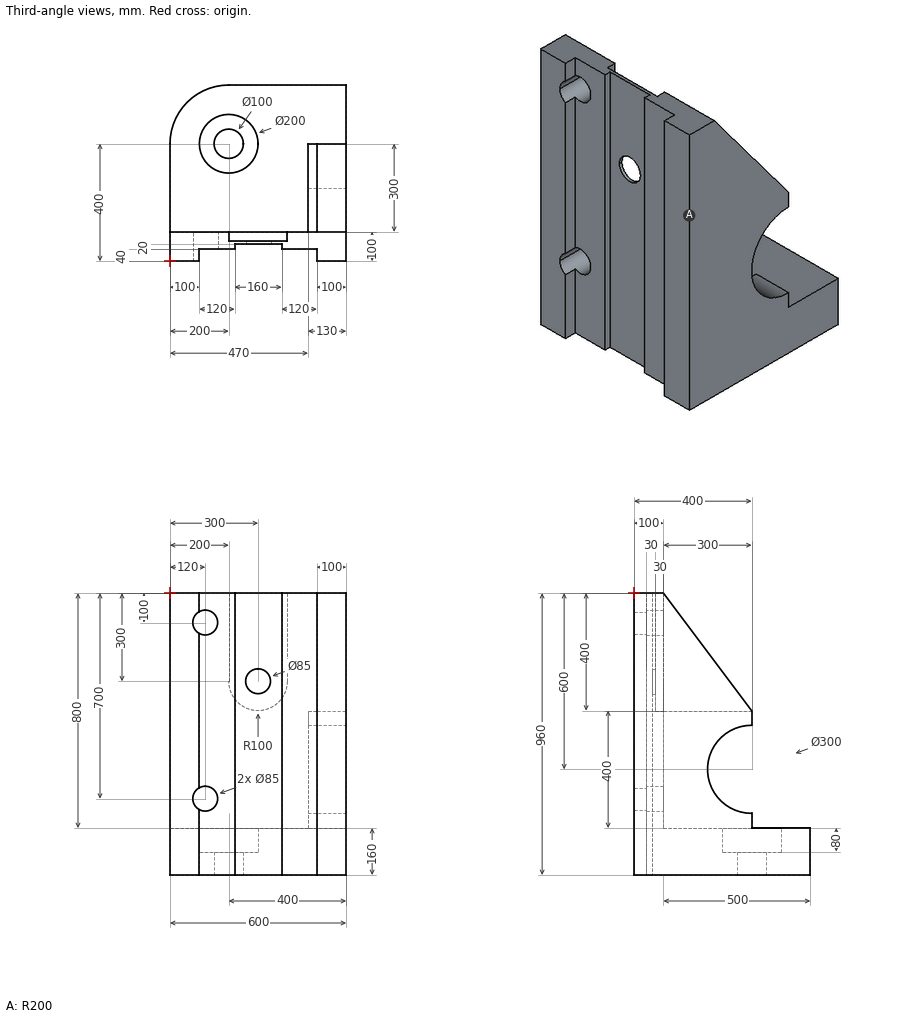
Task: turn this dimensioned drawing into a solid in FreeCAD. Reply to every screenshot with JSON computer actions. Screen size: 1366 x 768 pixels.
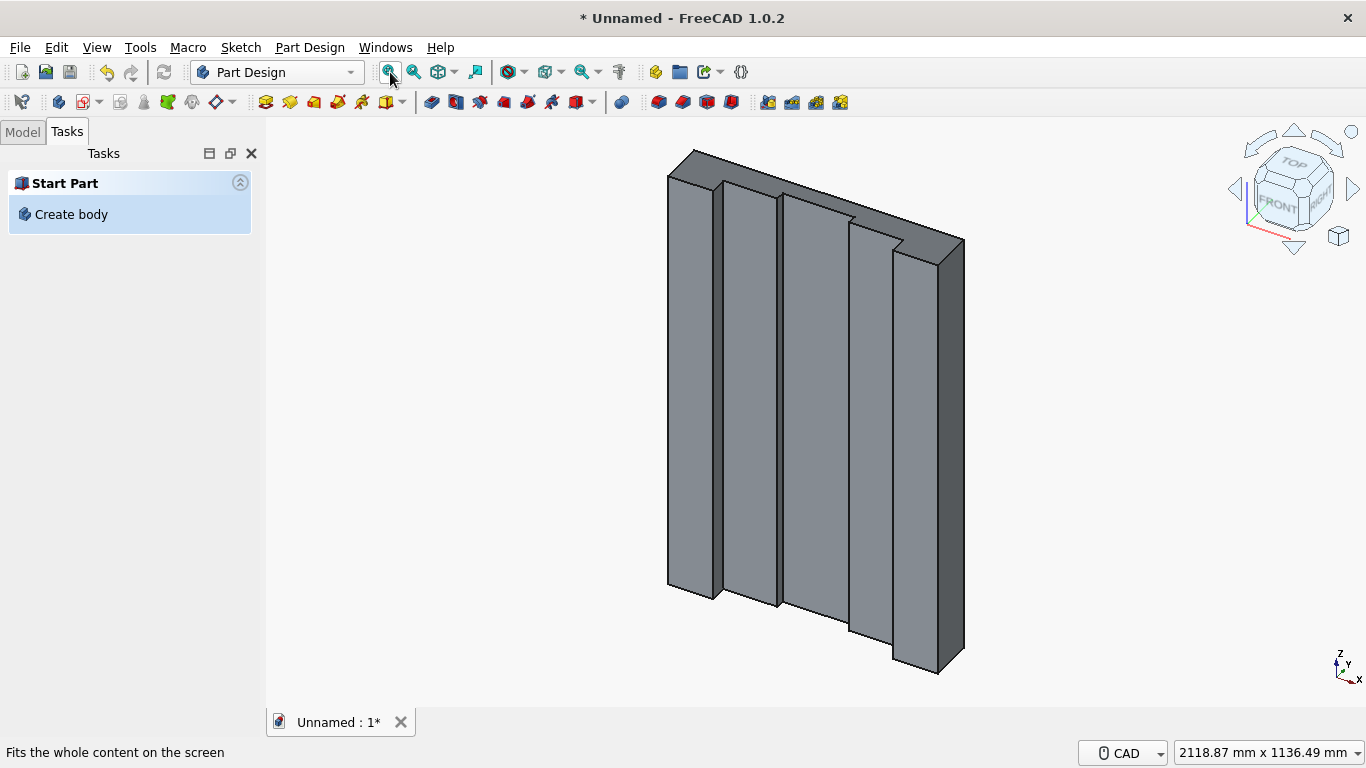
{"action": "key", "text": "4"}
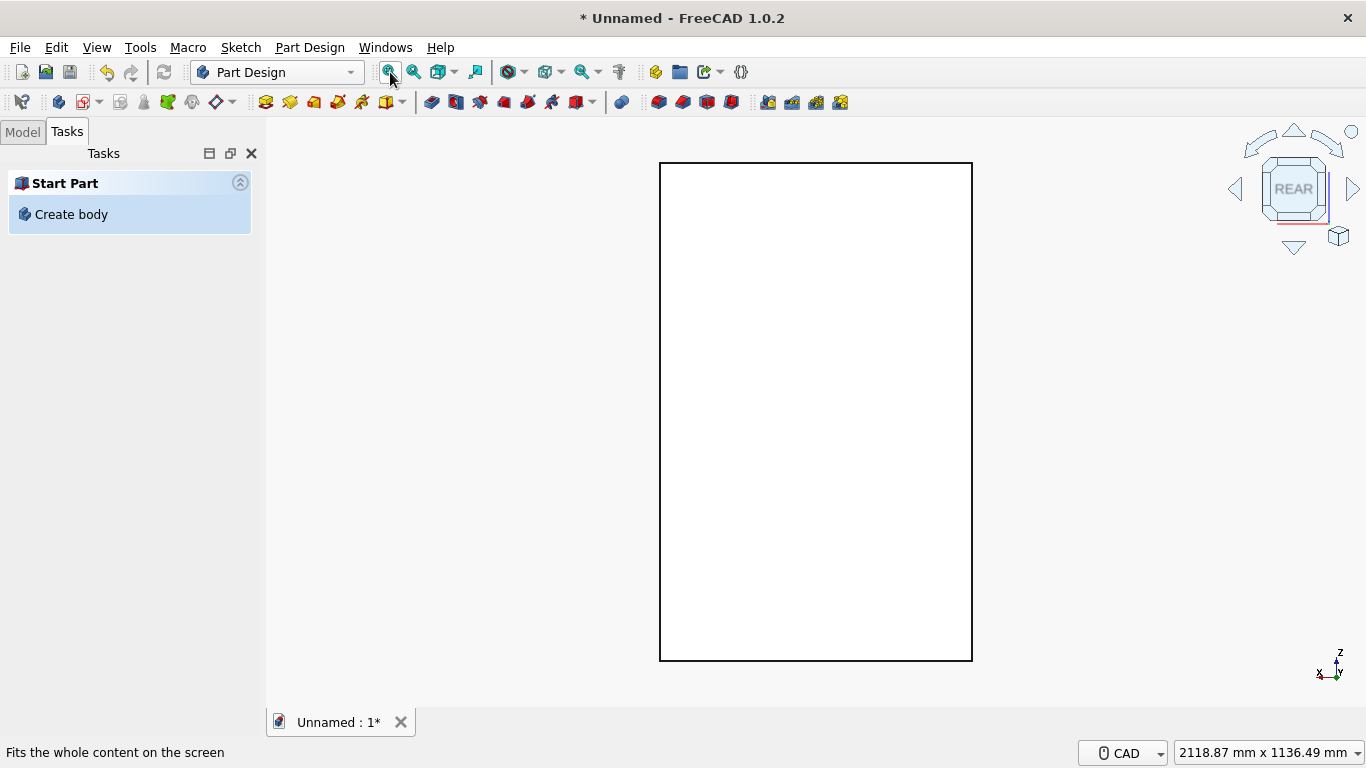
{"action": "left_click", "coordinate": [816, 340]}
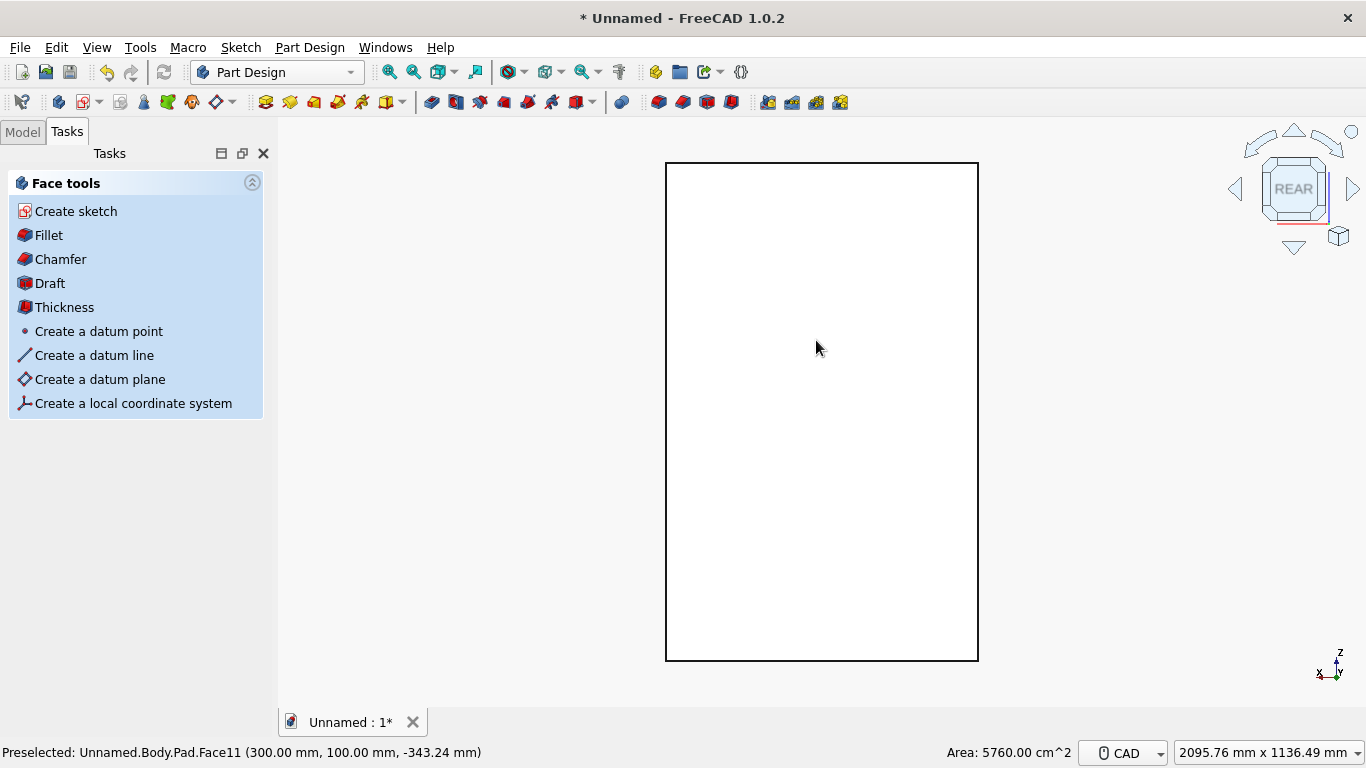
{"action": "left_click", "coordinate": [84, 102]}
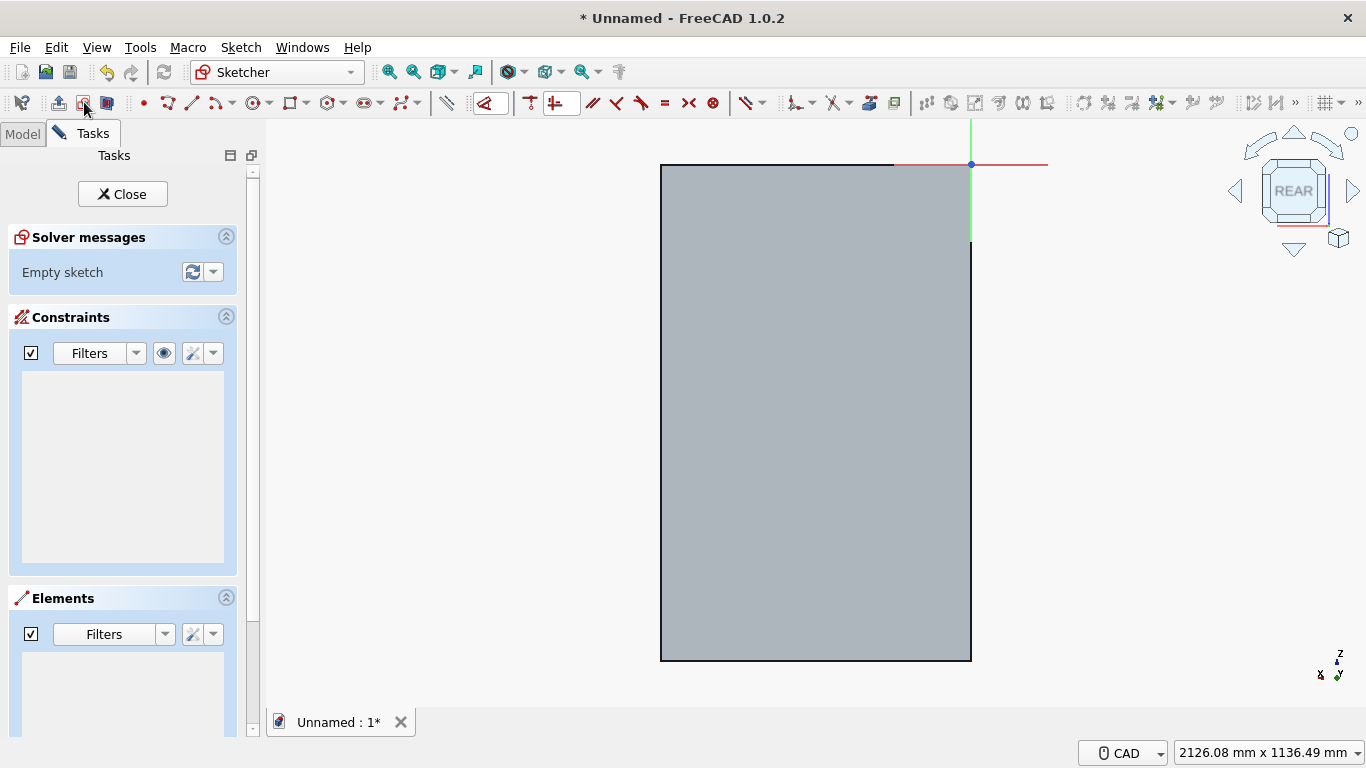
{"action": "scroll", "coordinate": [438, 413], "scroll_direction": "down", "scroll_amount": 1}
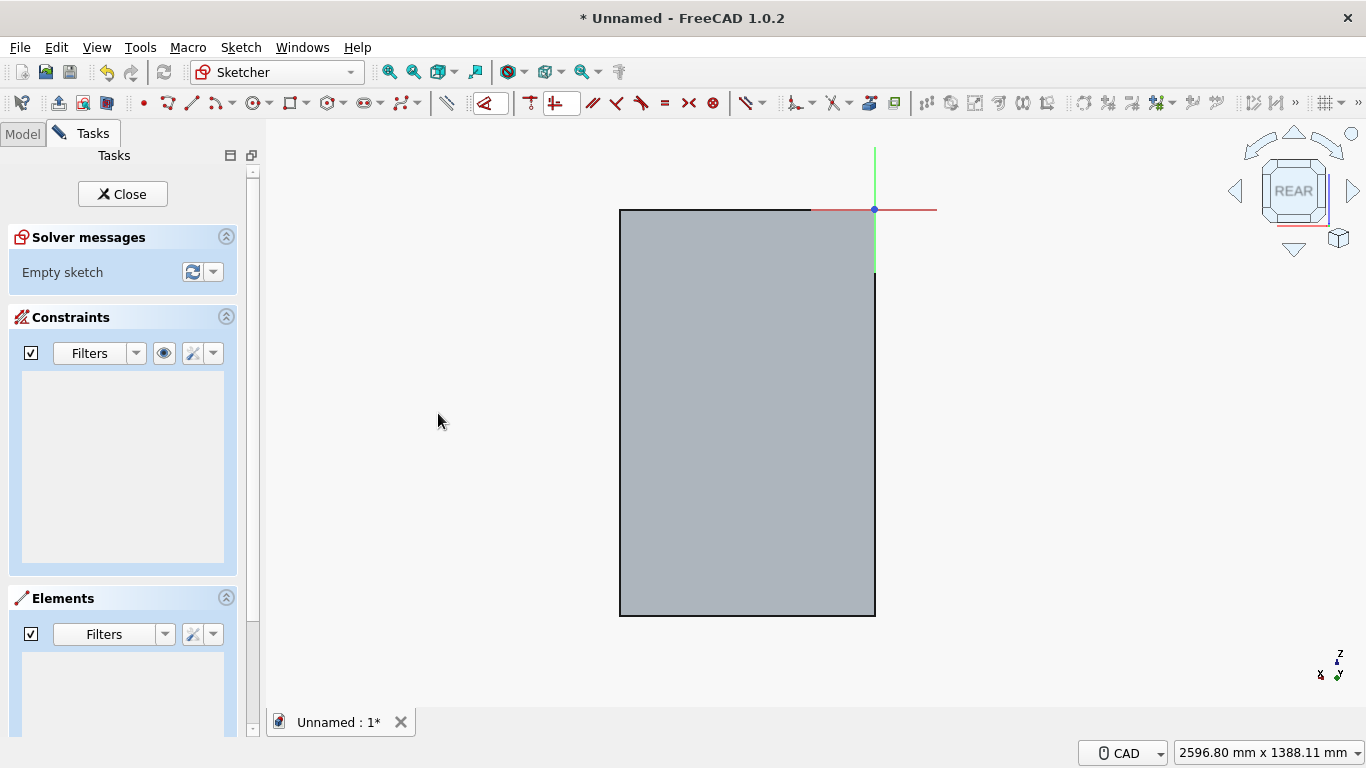
{"action": "left_click", "coordinate": [290, 104]}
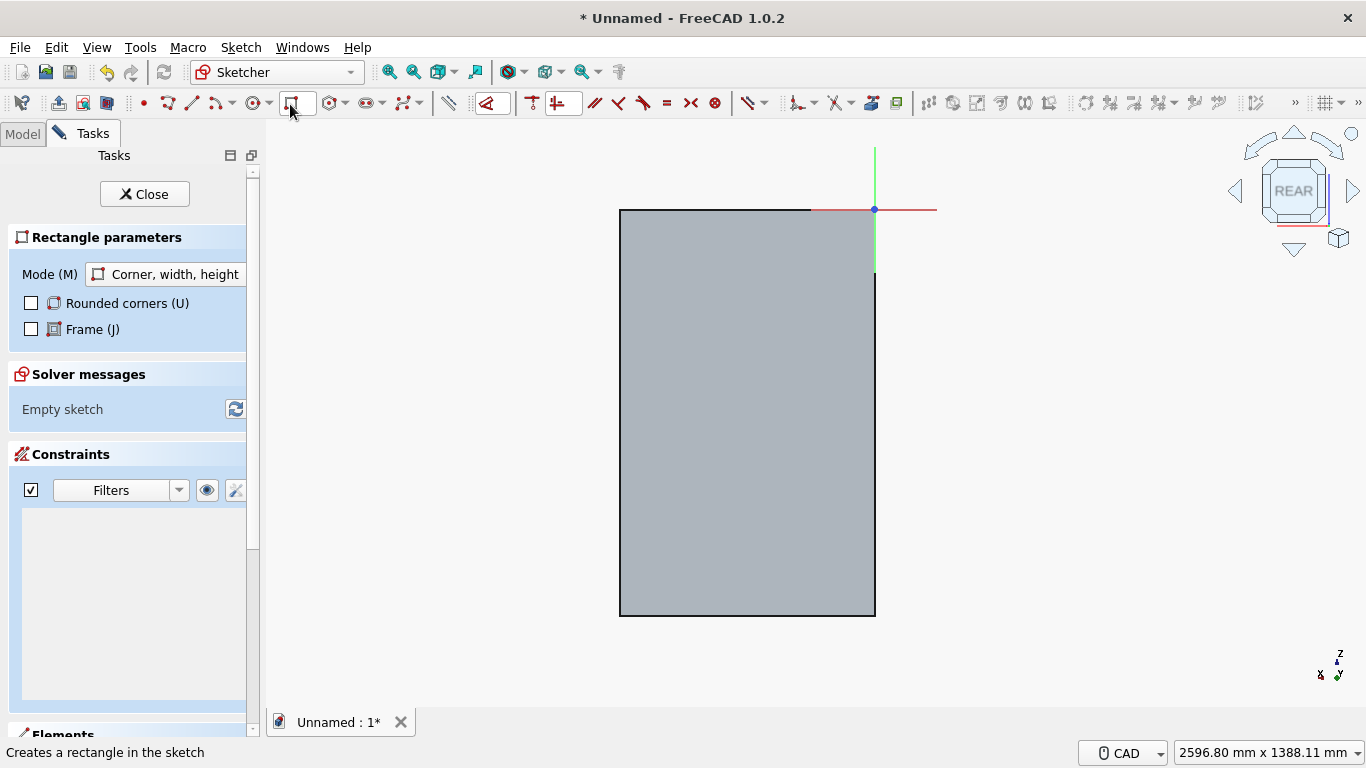
{"action": "left_click", "coordinate": [620, 549]}
{"action": "left_click", "coordinate": [875, 616]}
{"action": "key", "text": "Escape"}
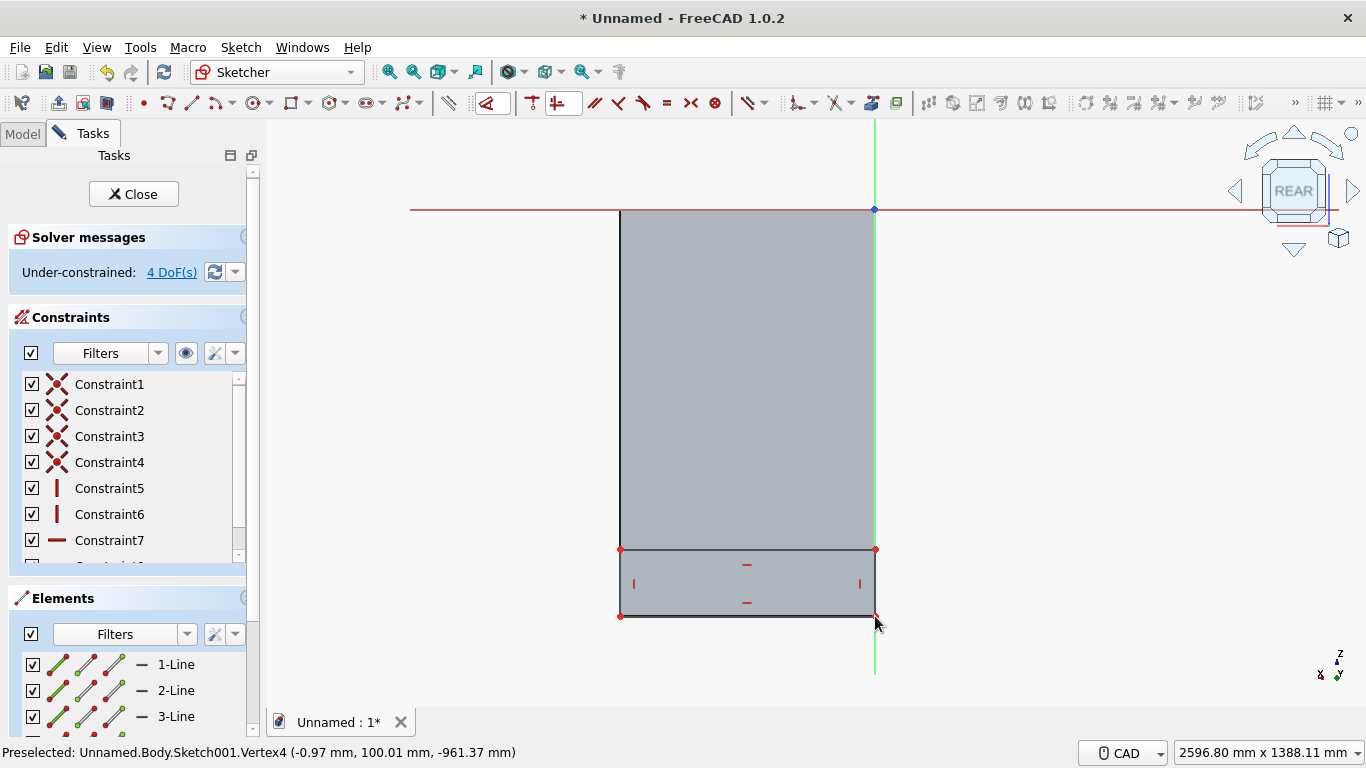
{"action": "left_click", "coordinate": [875, 617]}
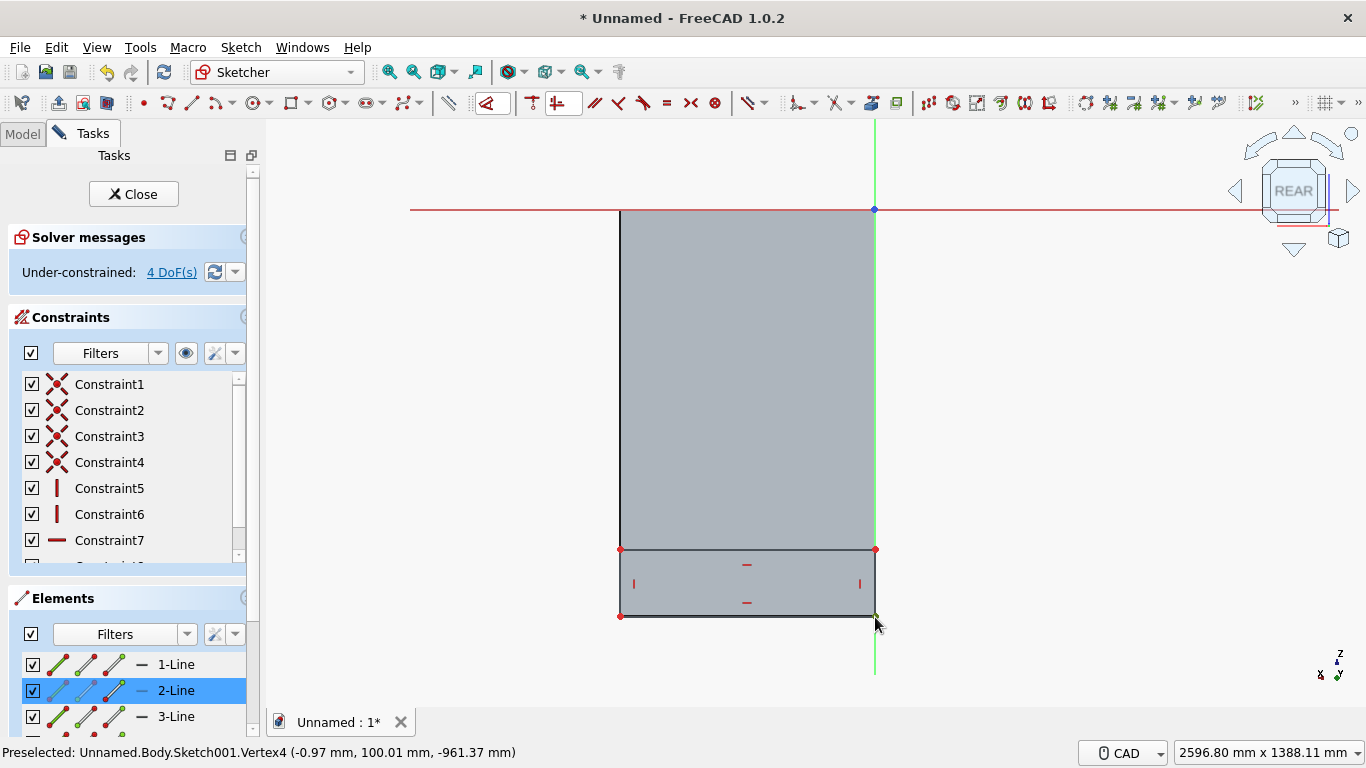
{"action": "left_click", "coordinate": [875, 489]}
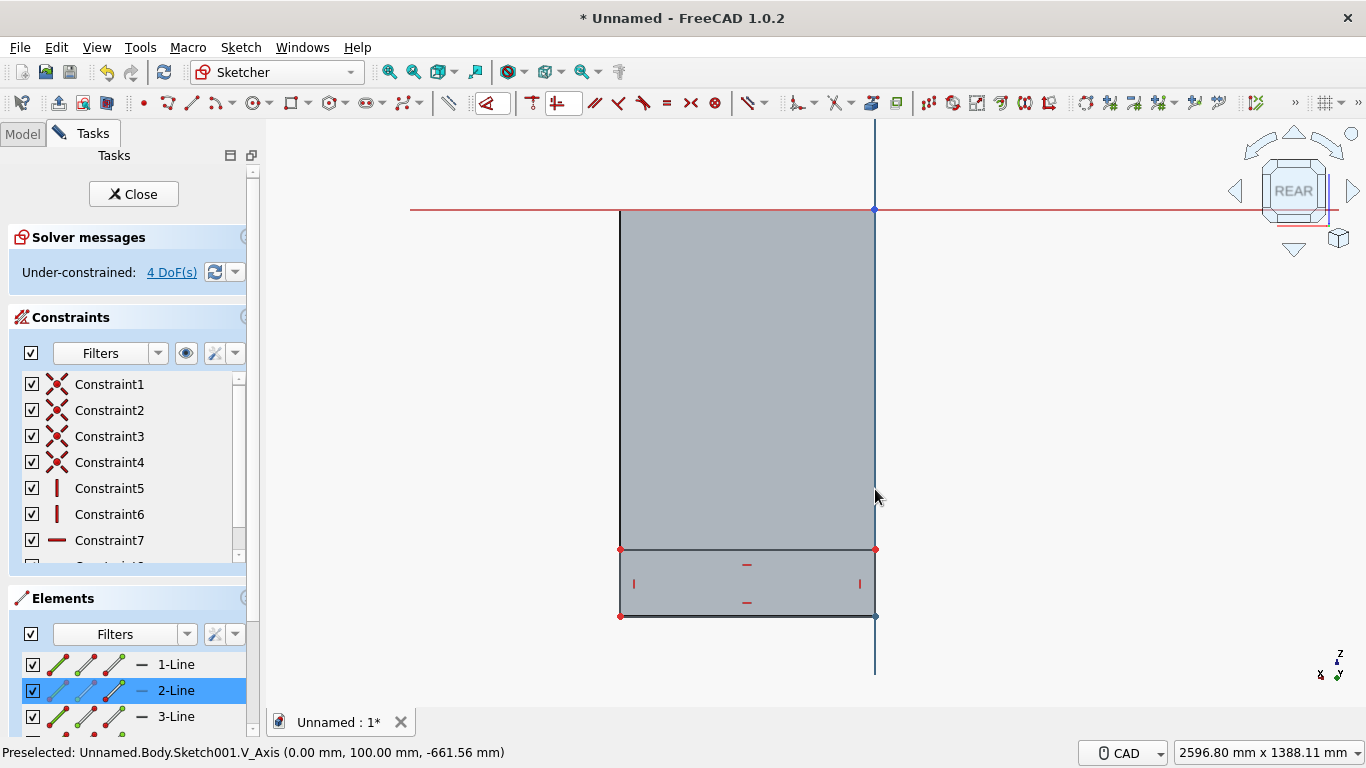
{"action": "left_click", "coordinate": [532, 104]}